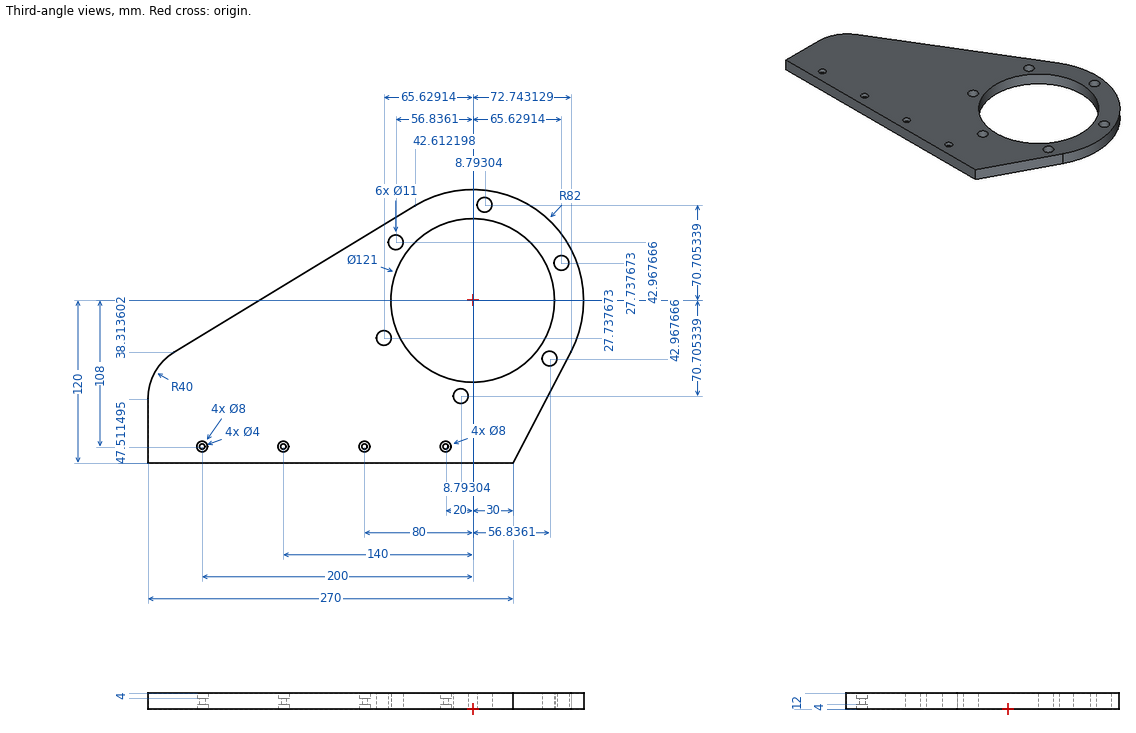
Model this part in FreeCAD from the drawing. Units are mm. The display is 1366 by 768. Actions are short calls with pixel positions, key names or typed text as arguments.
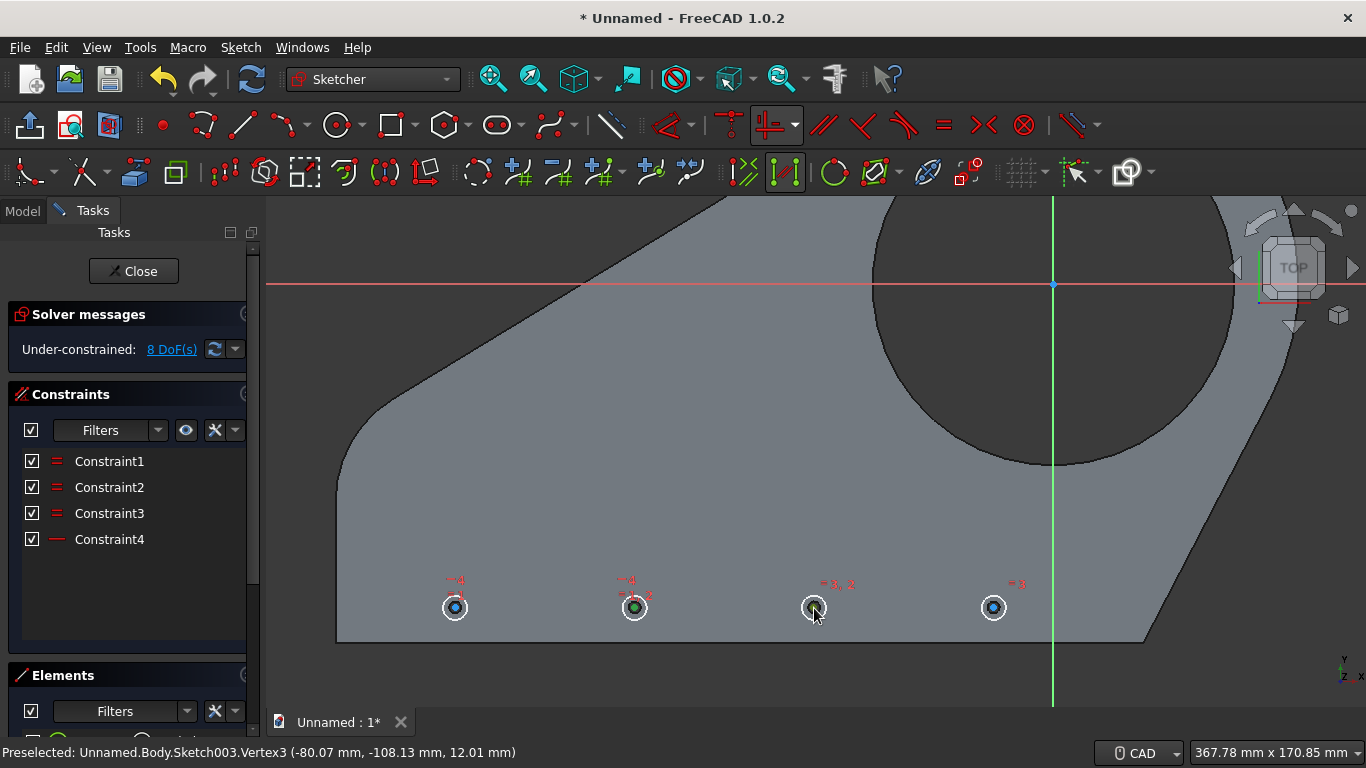
click(798, 126)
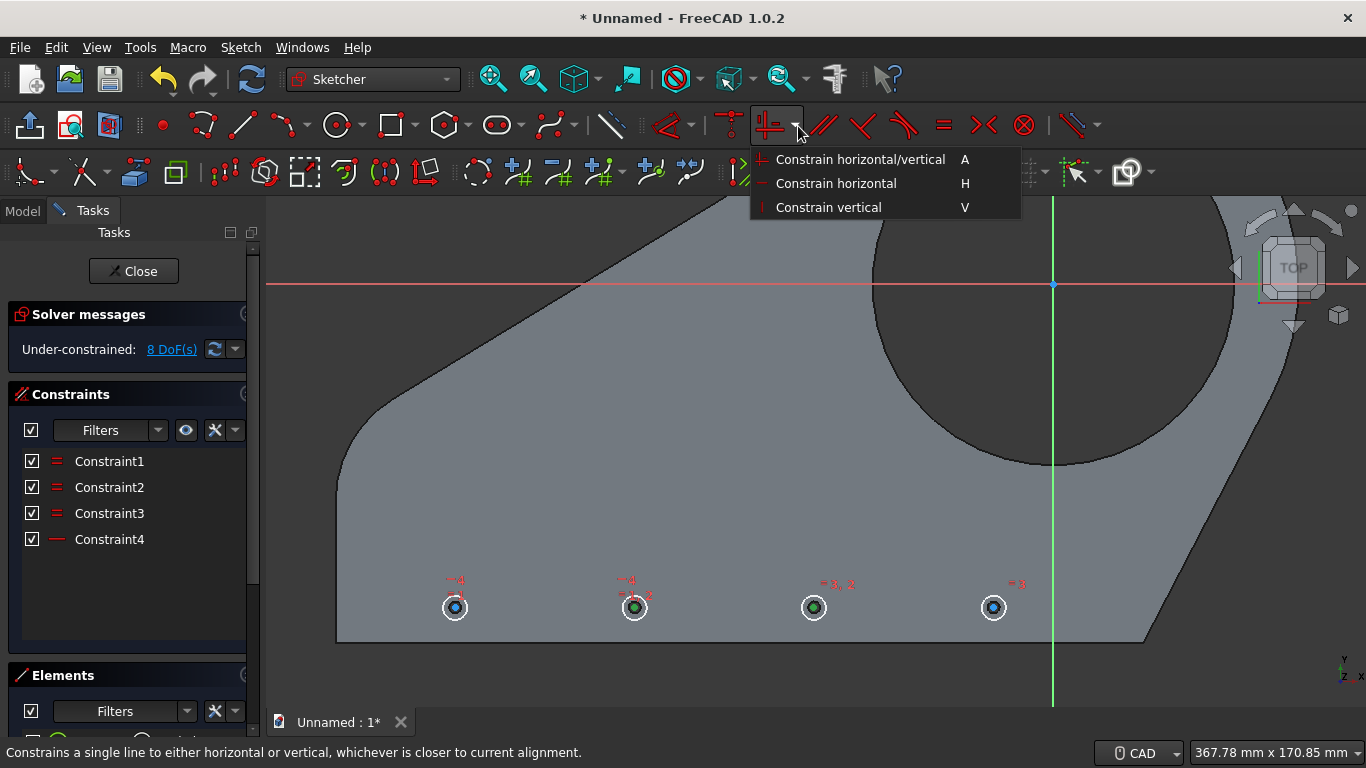
click(886, 183)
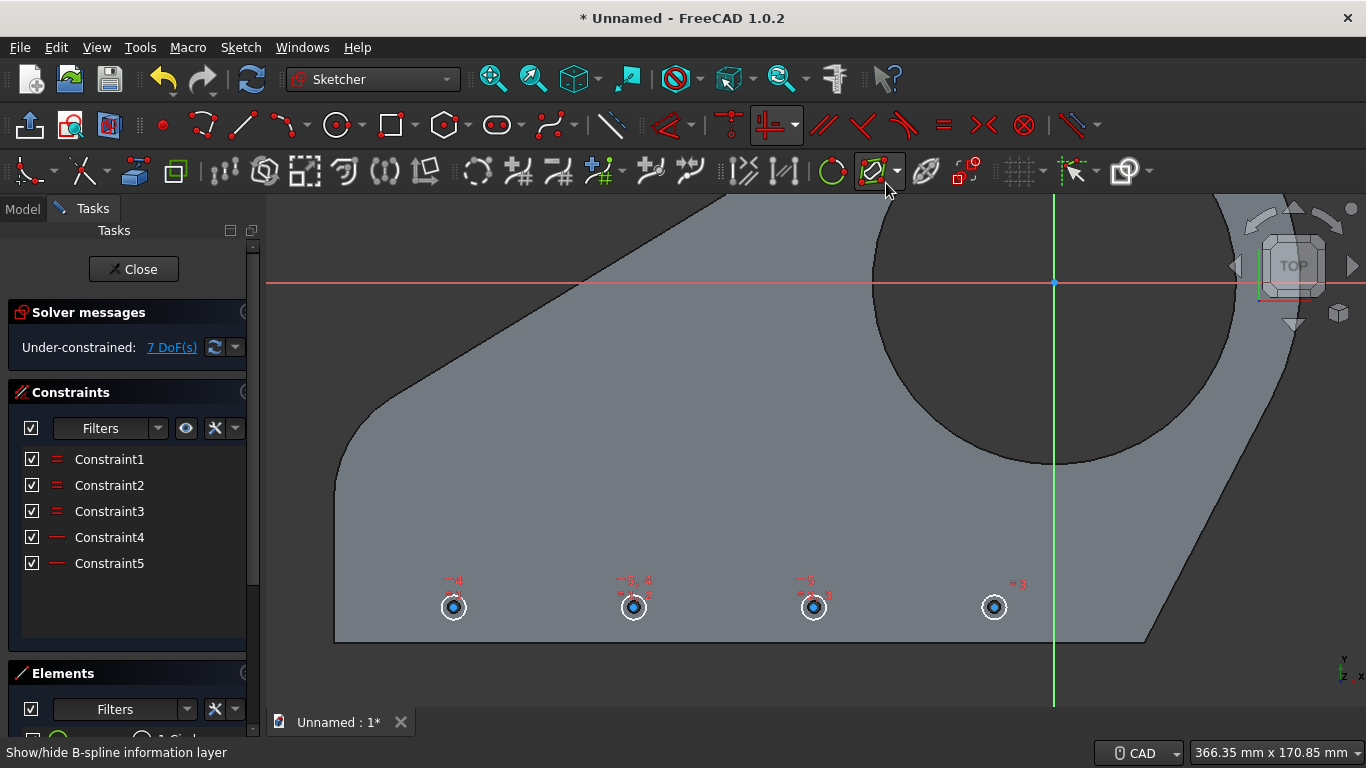
click(814, 608)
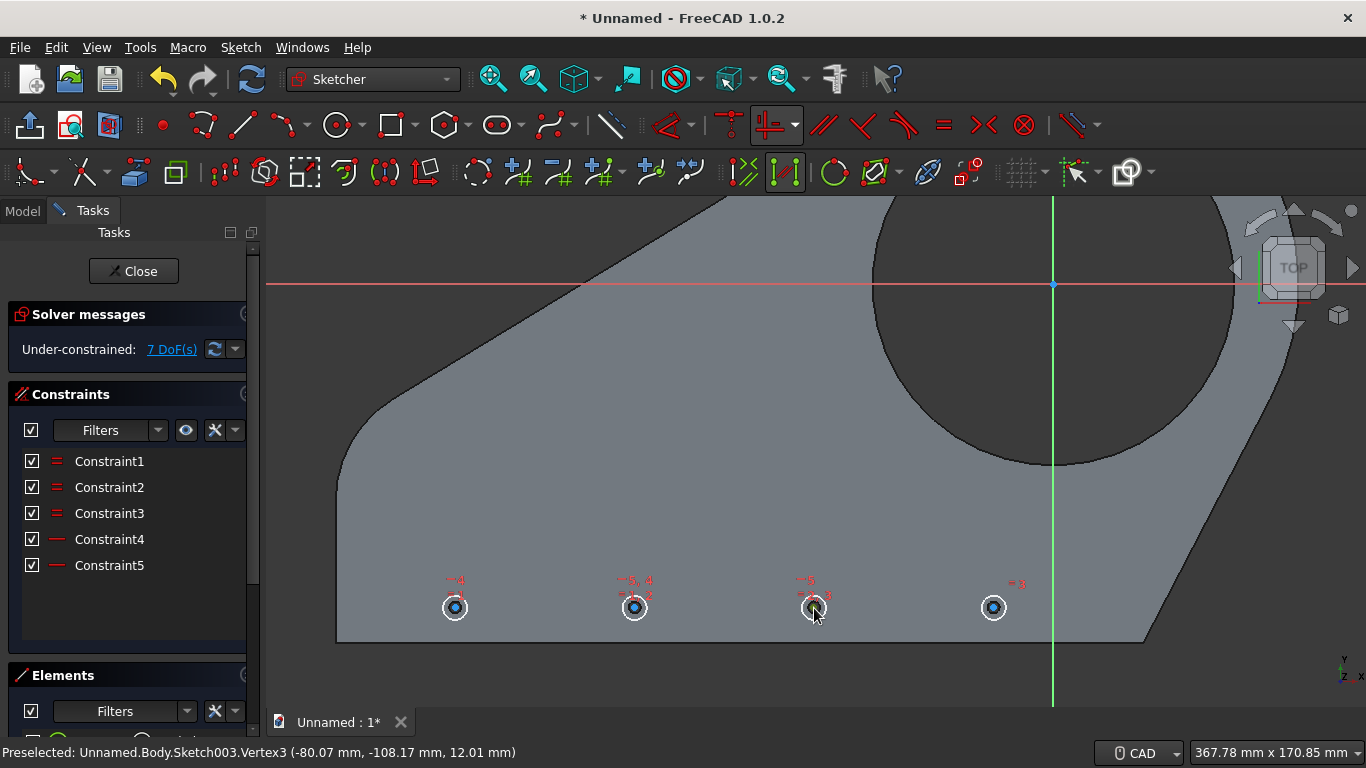
click(994, 608)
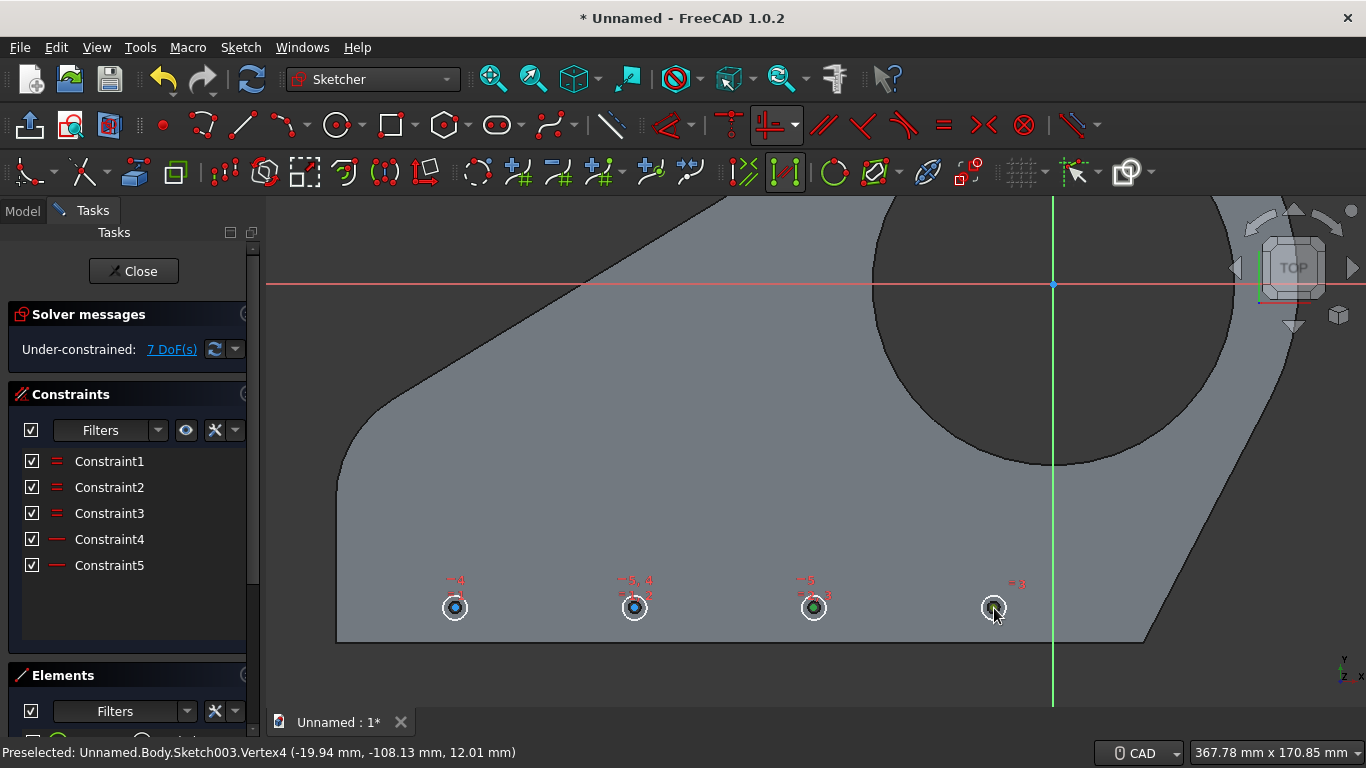
click(798, 126)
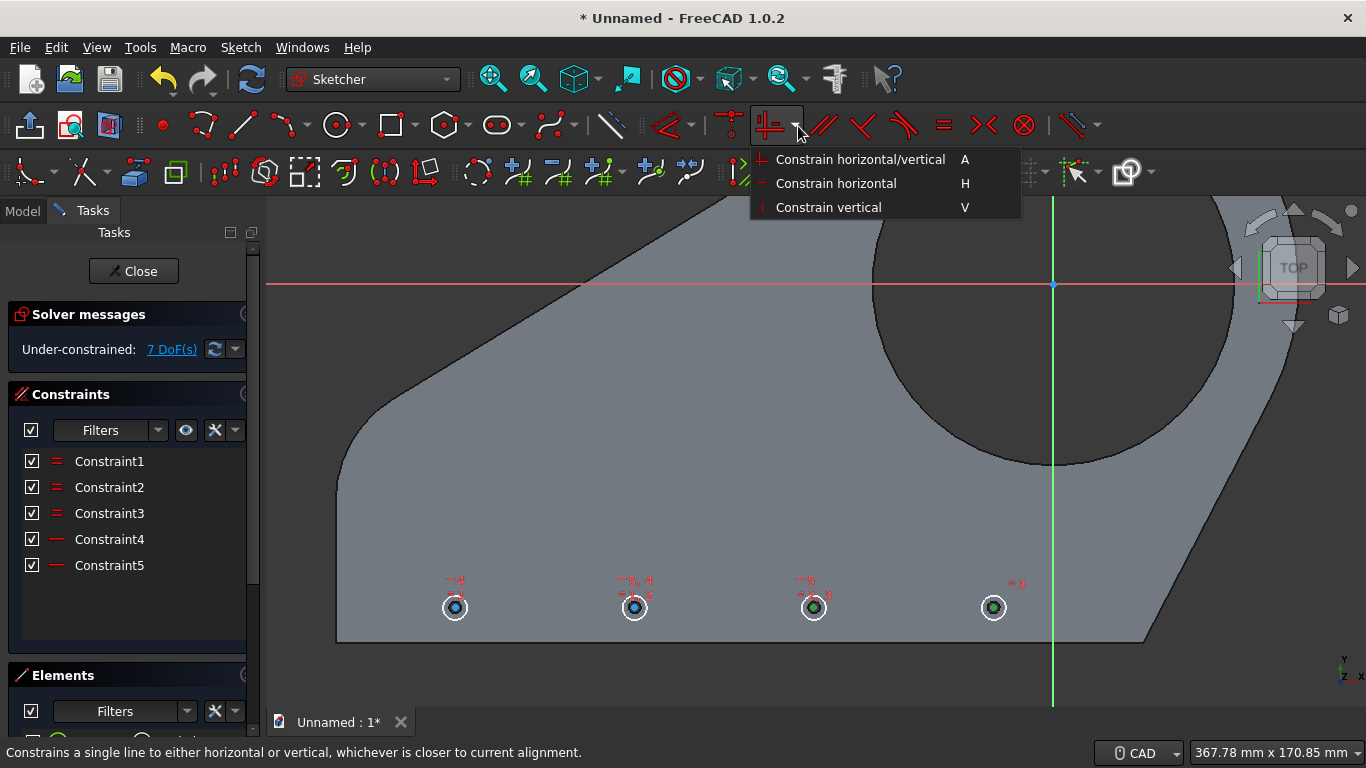
click(886, 183)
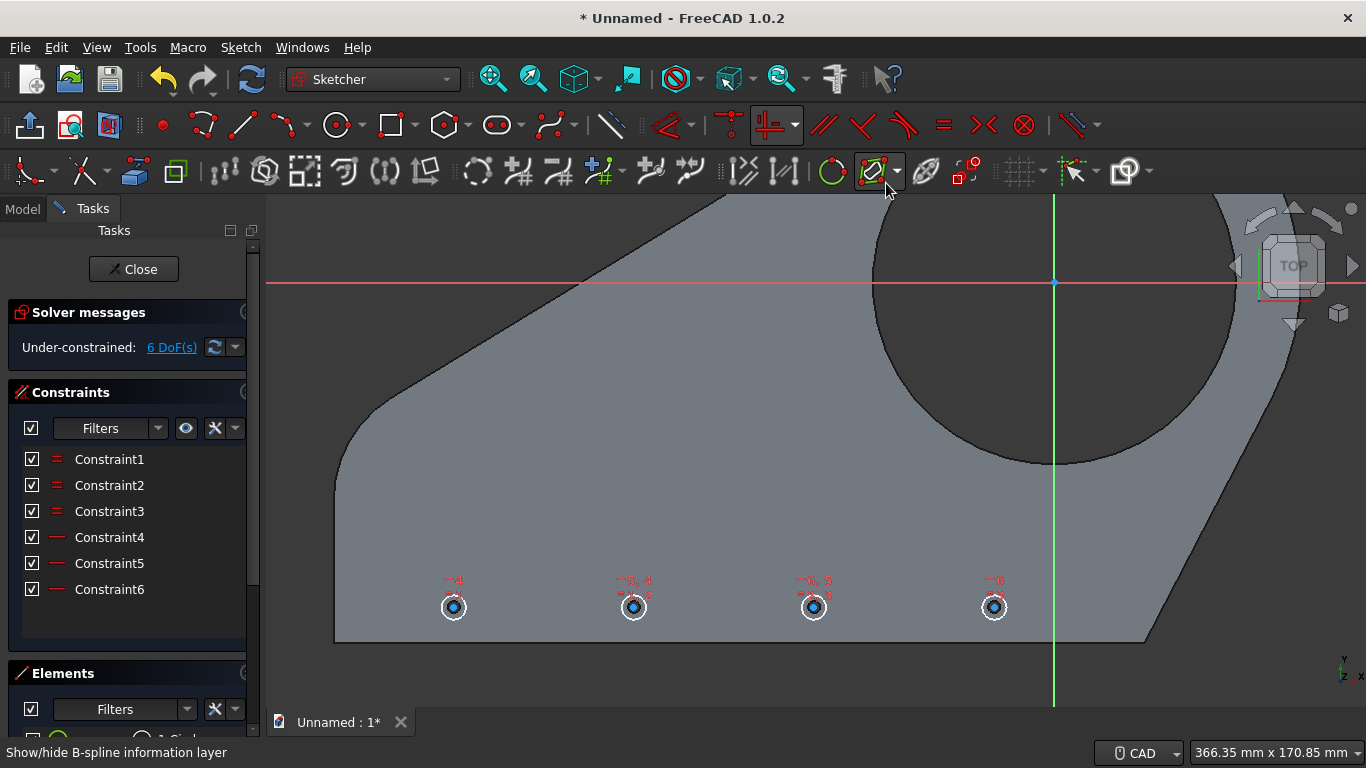
click(666, 126)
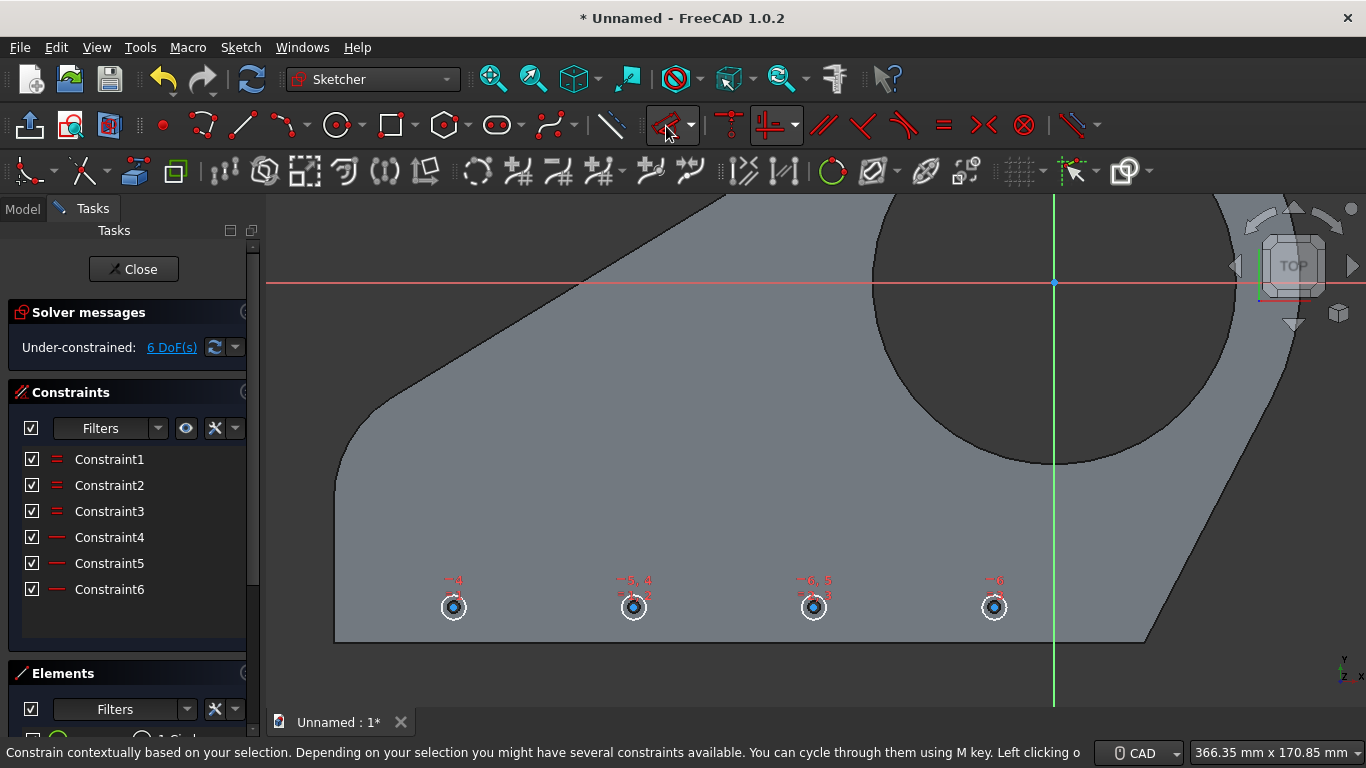
scroll(462, 599, up, 3)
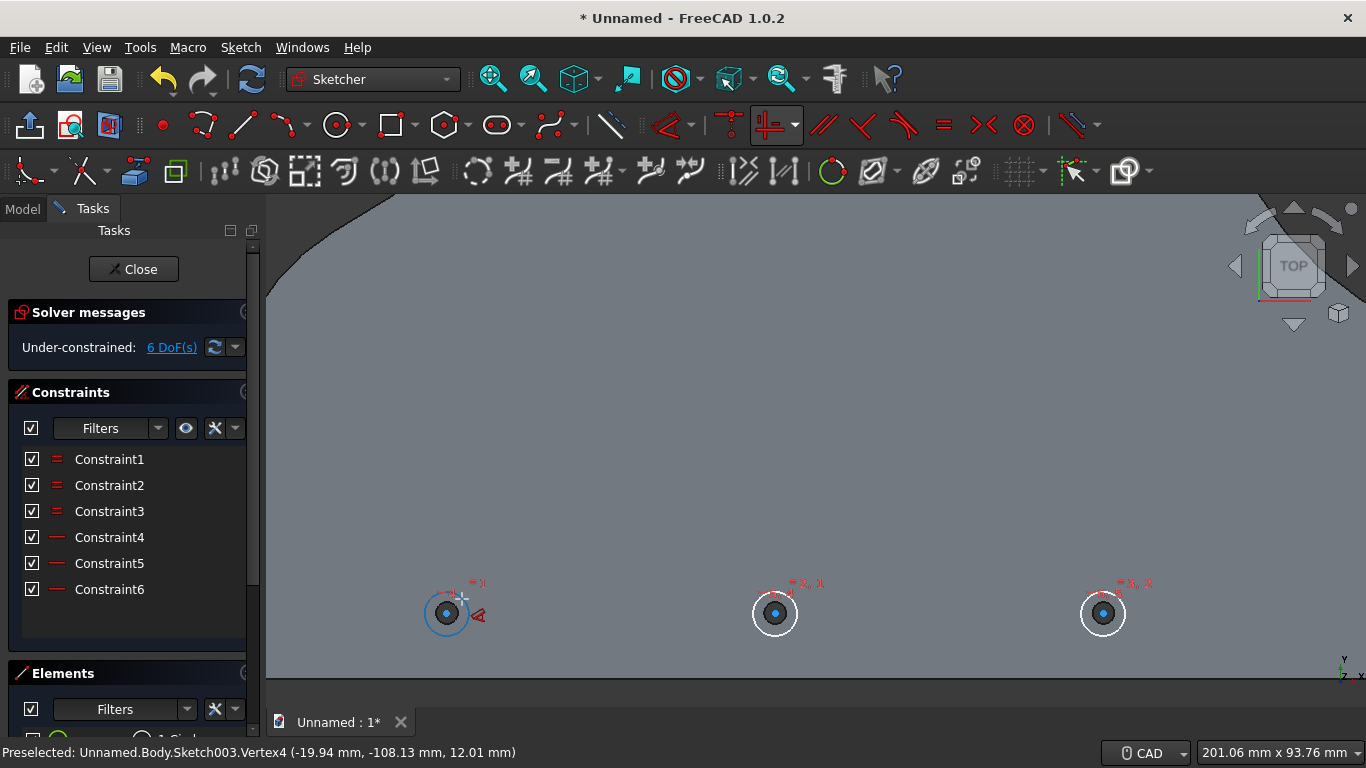
click(462, 598)
click(484, 575)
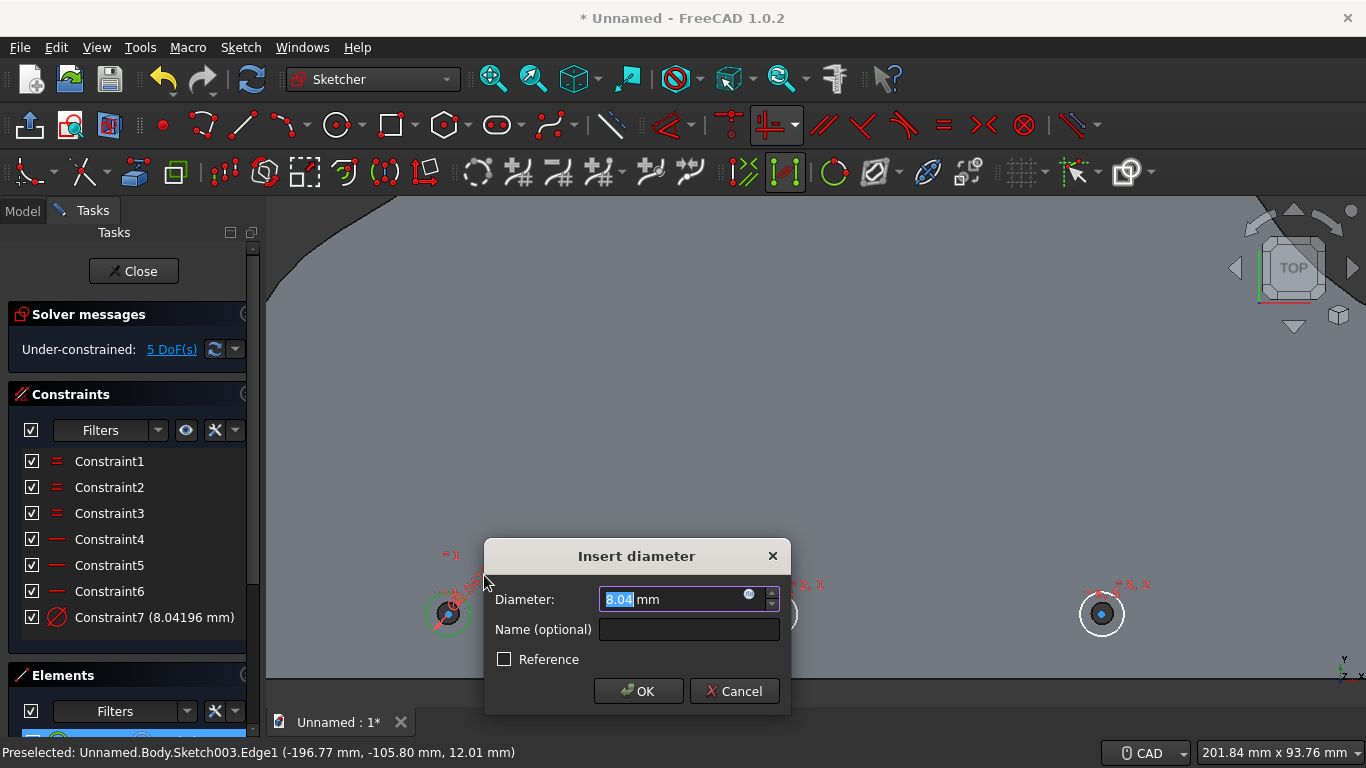
text(8)
key(Return)